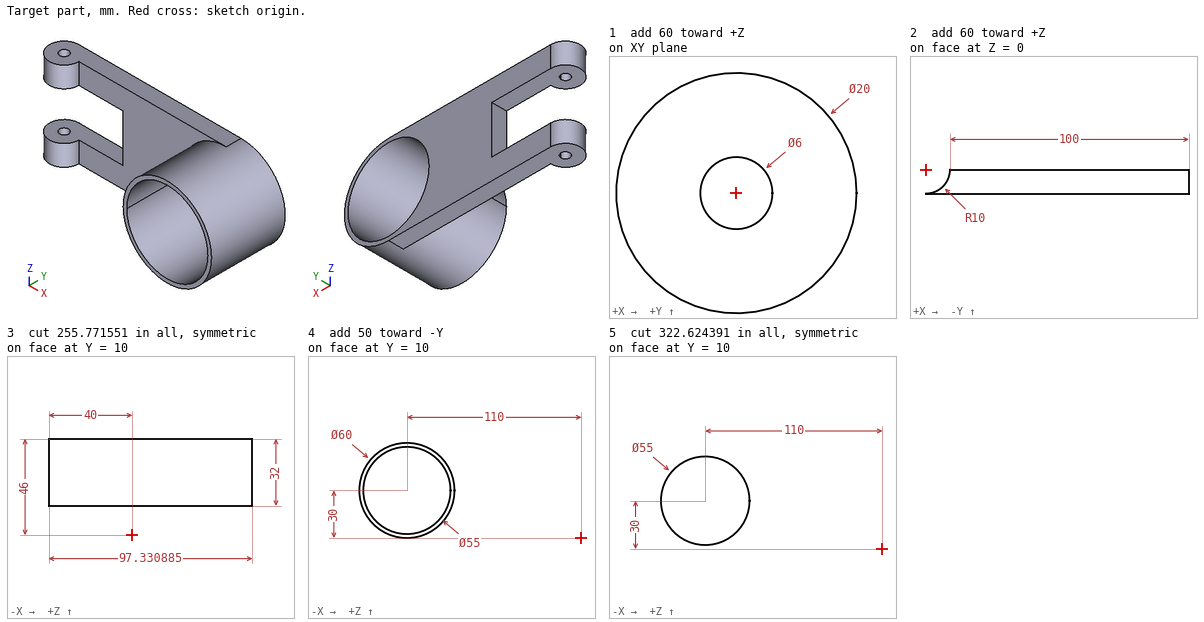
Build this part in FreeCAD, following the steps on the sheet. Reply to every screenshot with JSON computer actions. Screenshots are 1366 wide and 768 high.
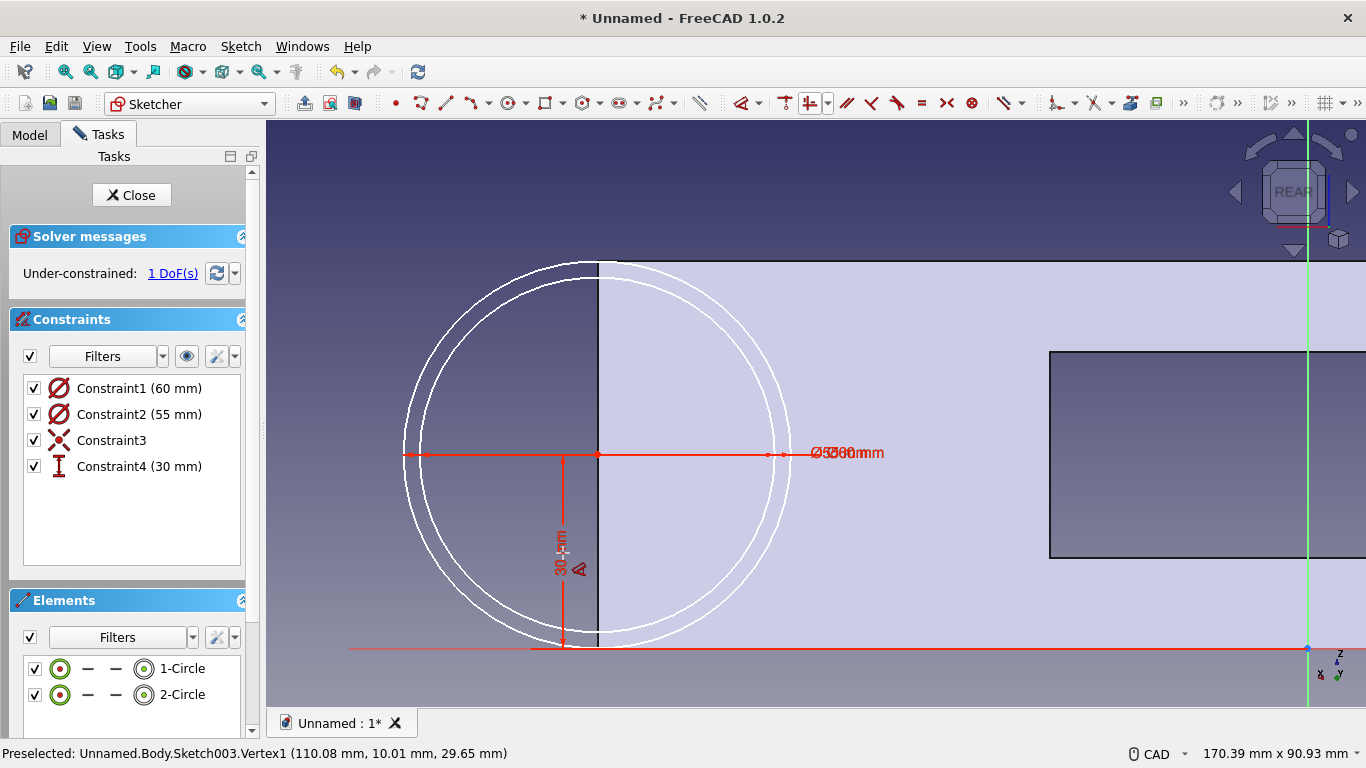
{"action": "left_click", "coordinate": [597, 455]}
{"action": "left_click", "coordinate": [899, 421]}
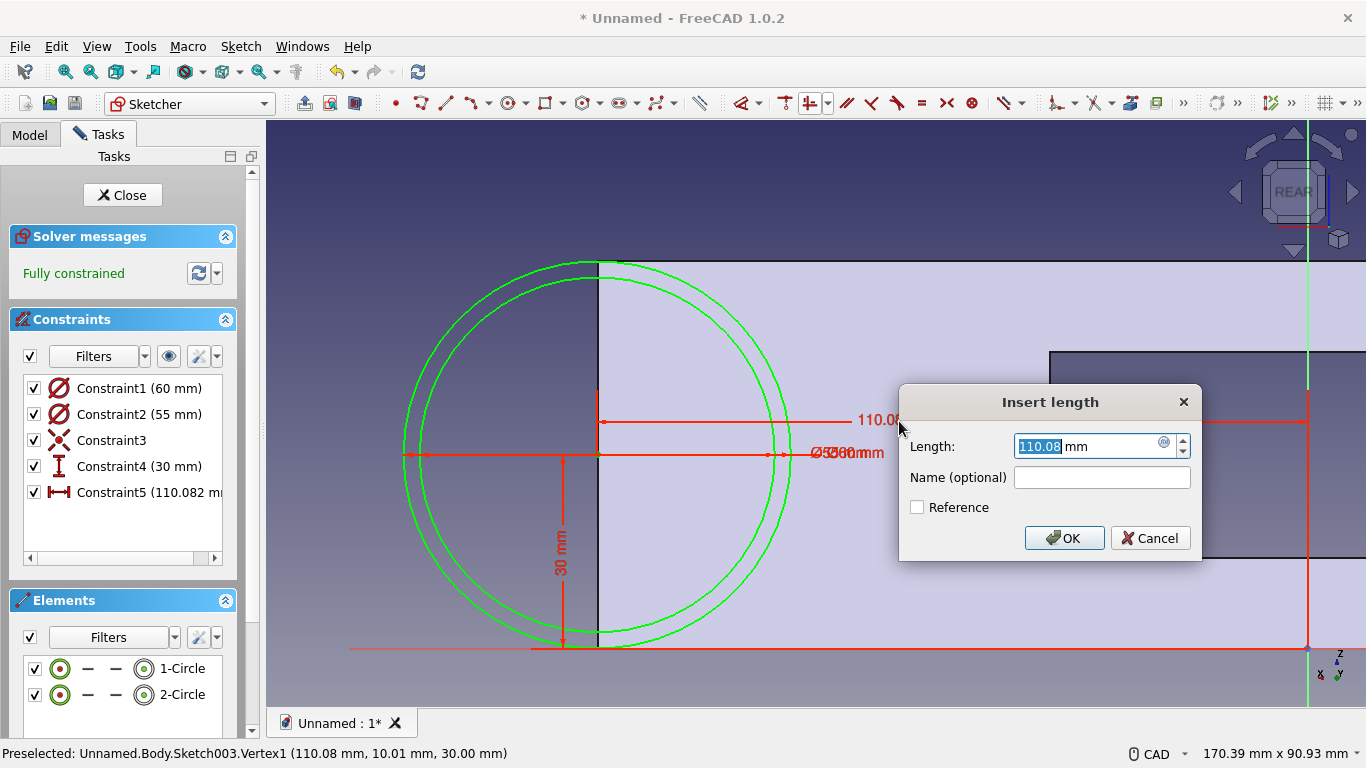
{"action": "type", "text": "110"}
{"action": "key", "text": "Return"}
{"action": "key", "text": "Escape"}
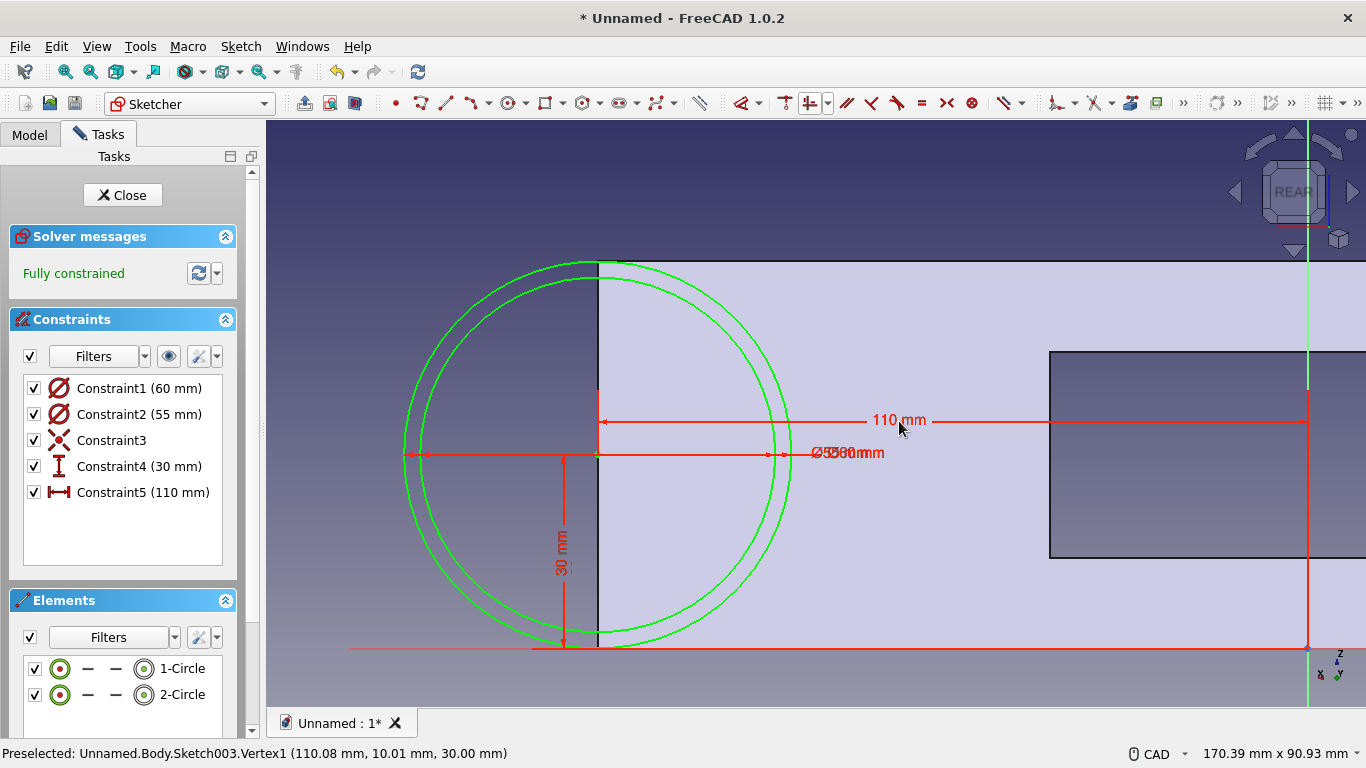
{"action": "left_click", "coordinate": [123, 195]}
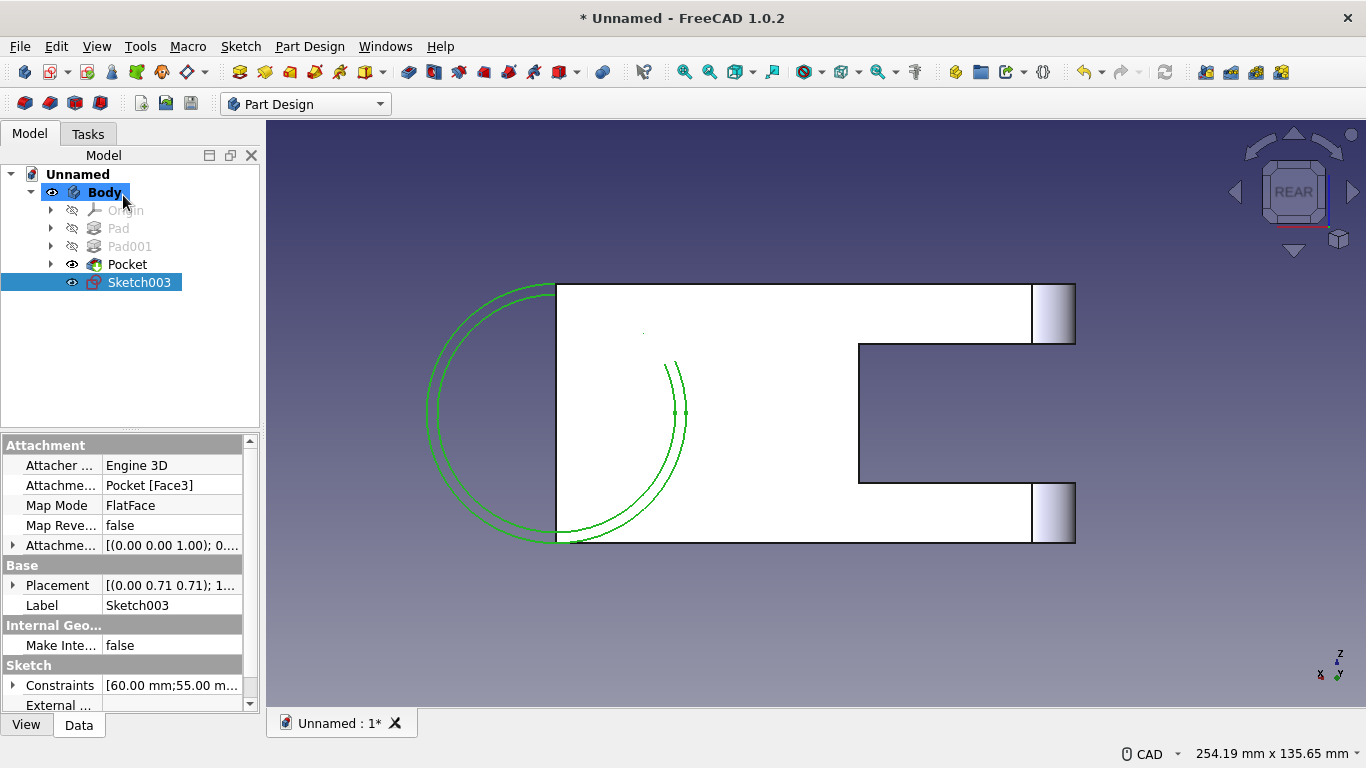
{"action": "left_click", "coordinate": [240, 72]}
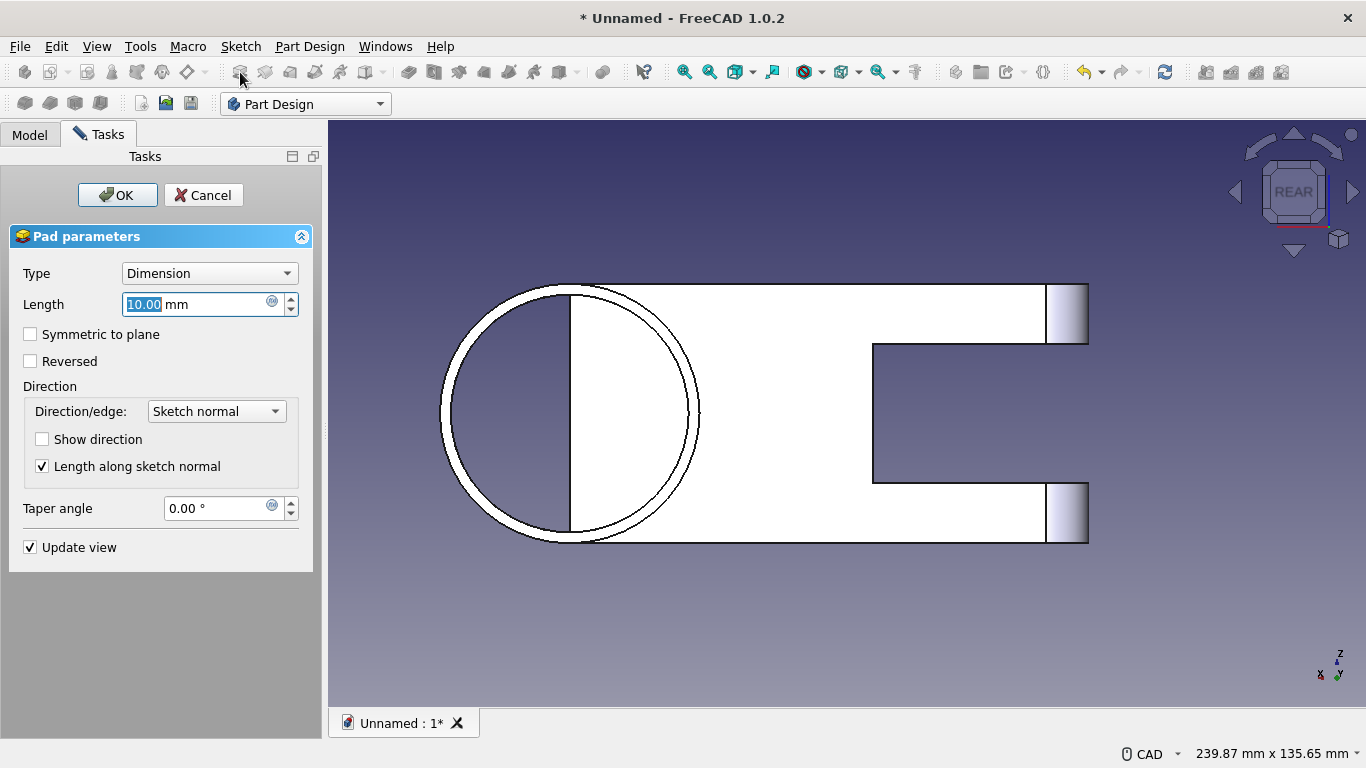
{"action": "type", "text": "50"}
{"action": "key", "text": "Tab"}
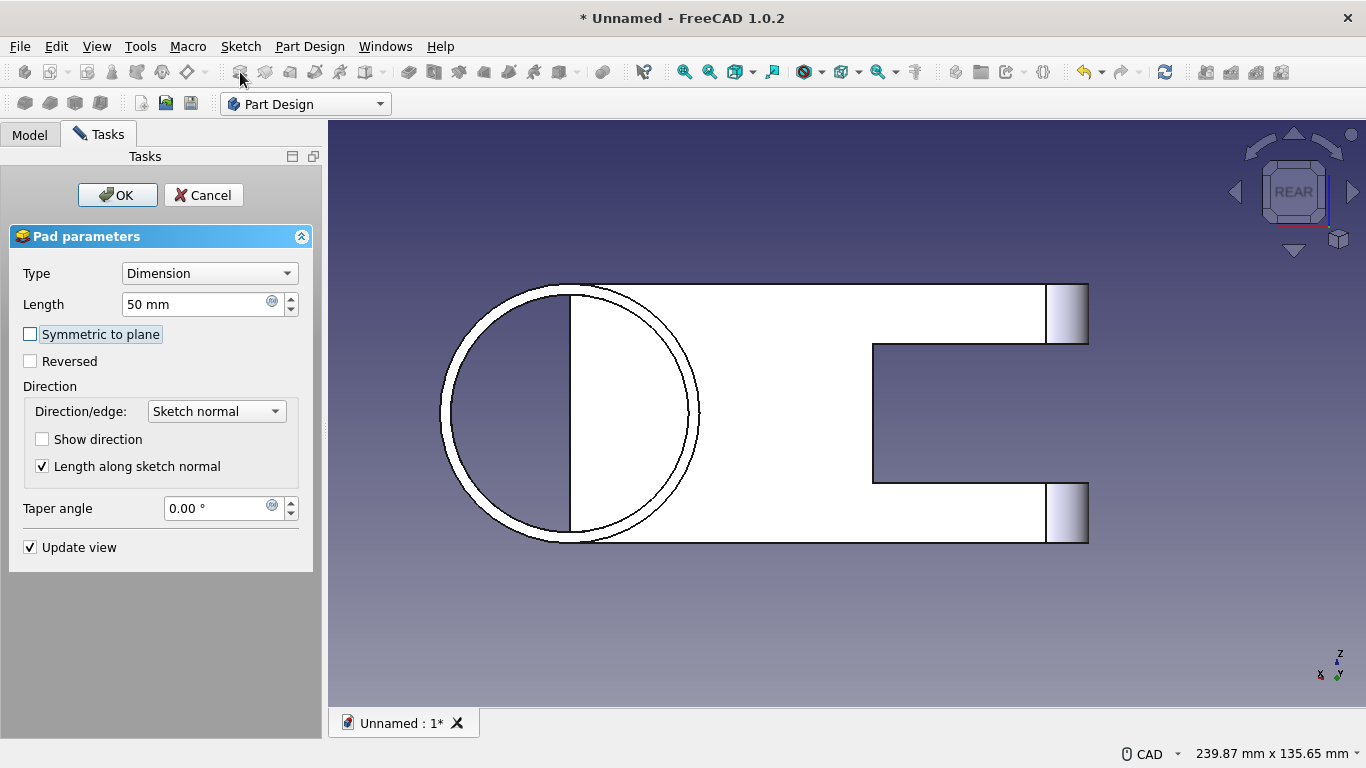
{"action": "left_click", "coordinate": [31, 361]}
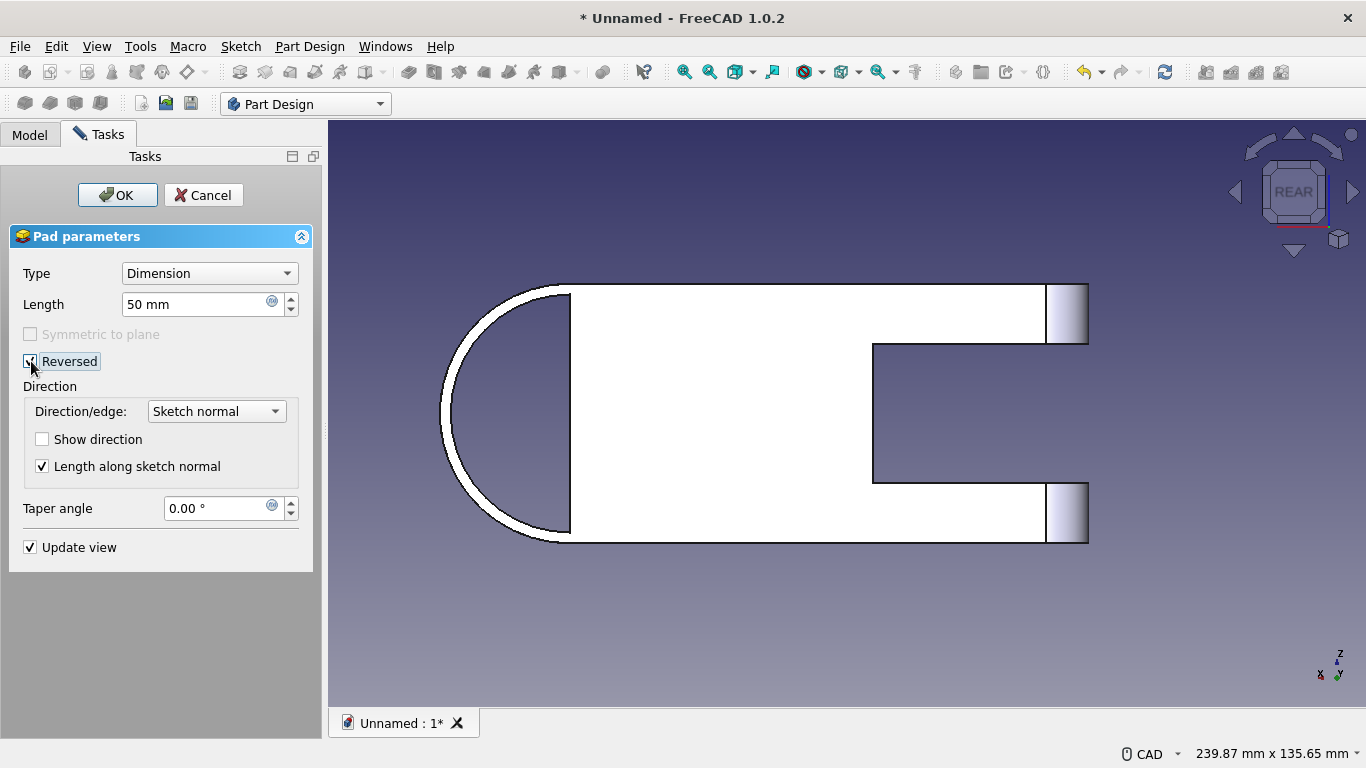
{"action": "left_click", "coordinate": [118, 195]}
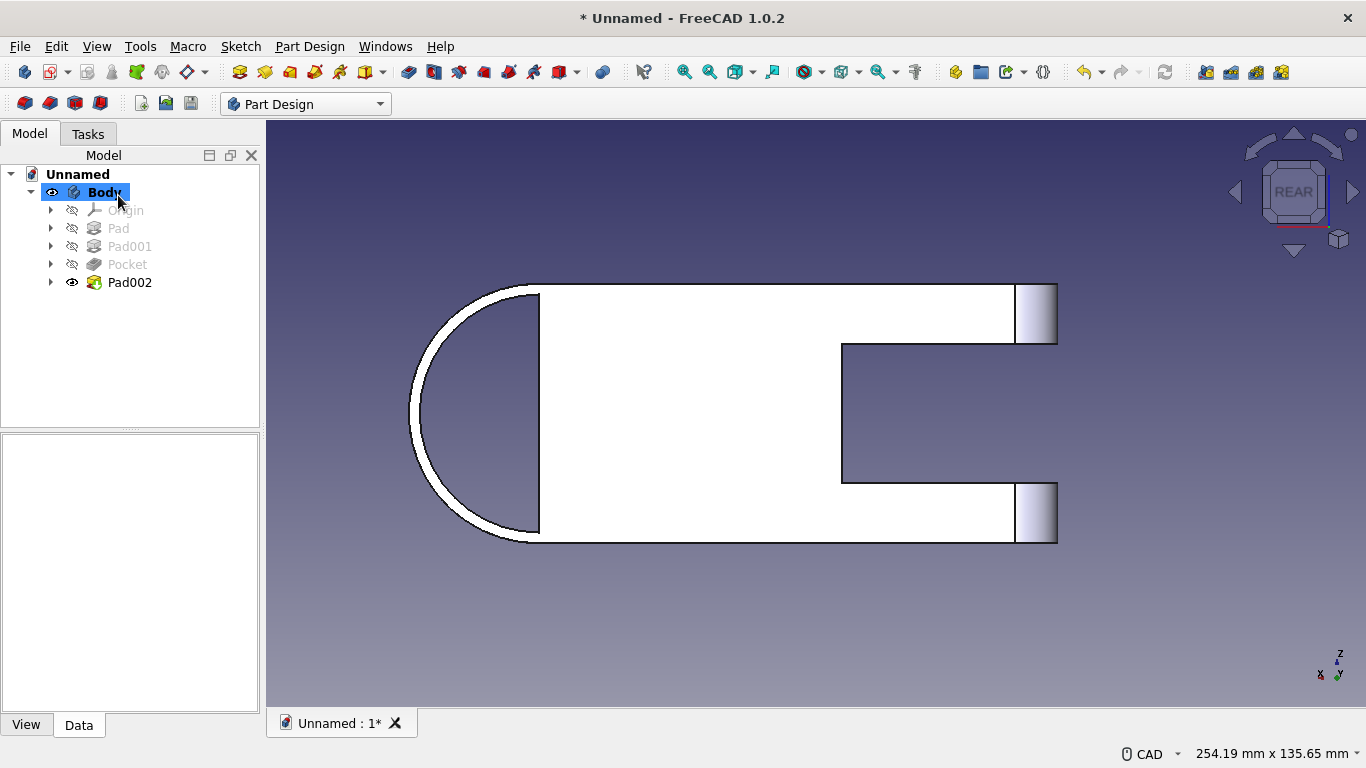
{"action": "left_click", "coordinate": [712, 412]}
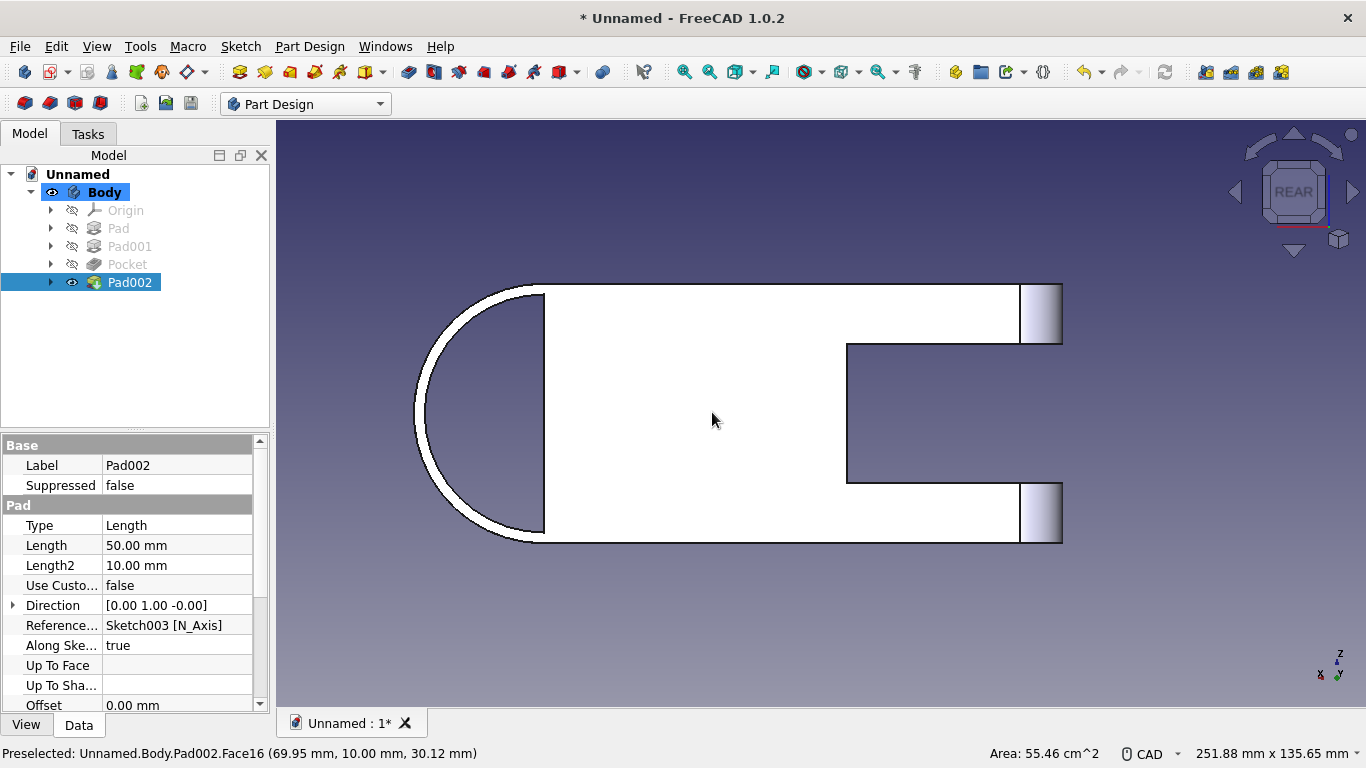
{"action": "left_click", "coordinate": [50, 72]}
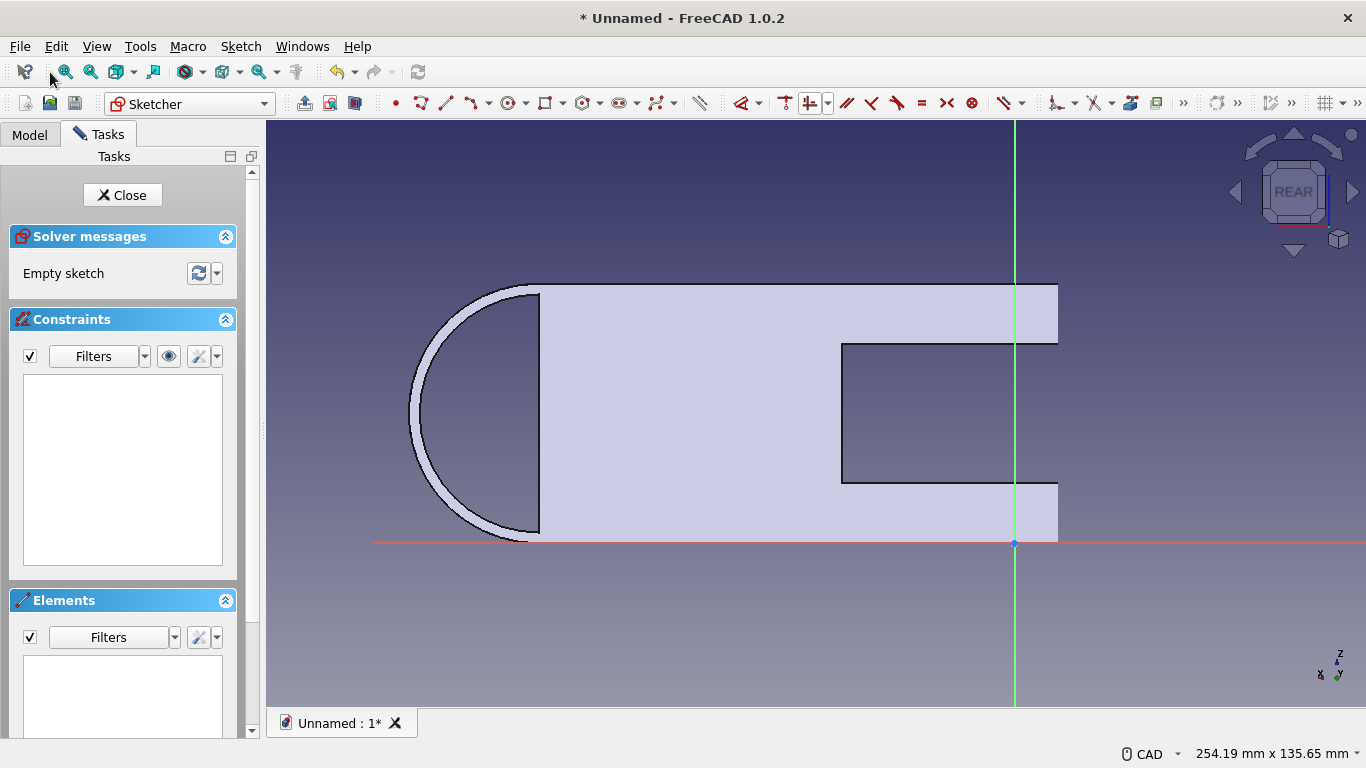
{"action": "scroll", "coordinate": [294, 414], "scroll_direction": "up", "scroll_amount": 2}